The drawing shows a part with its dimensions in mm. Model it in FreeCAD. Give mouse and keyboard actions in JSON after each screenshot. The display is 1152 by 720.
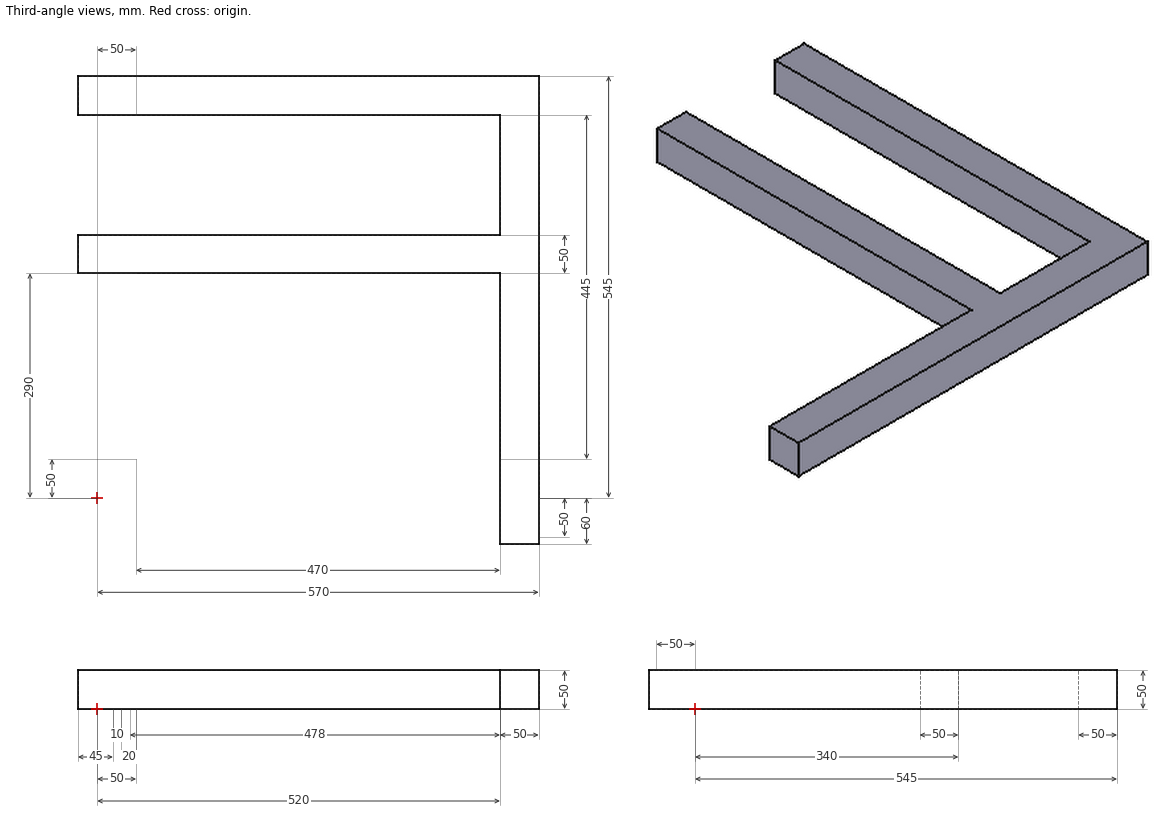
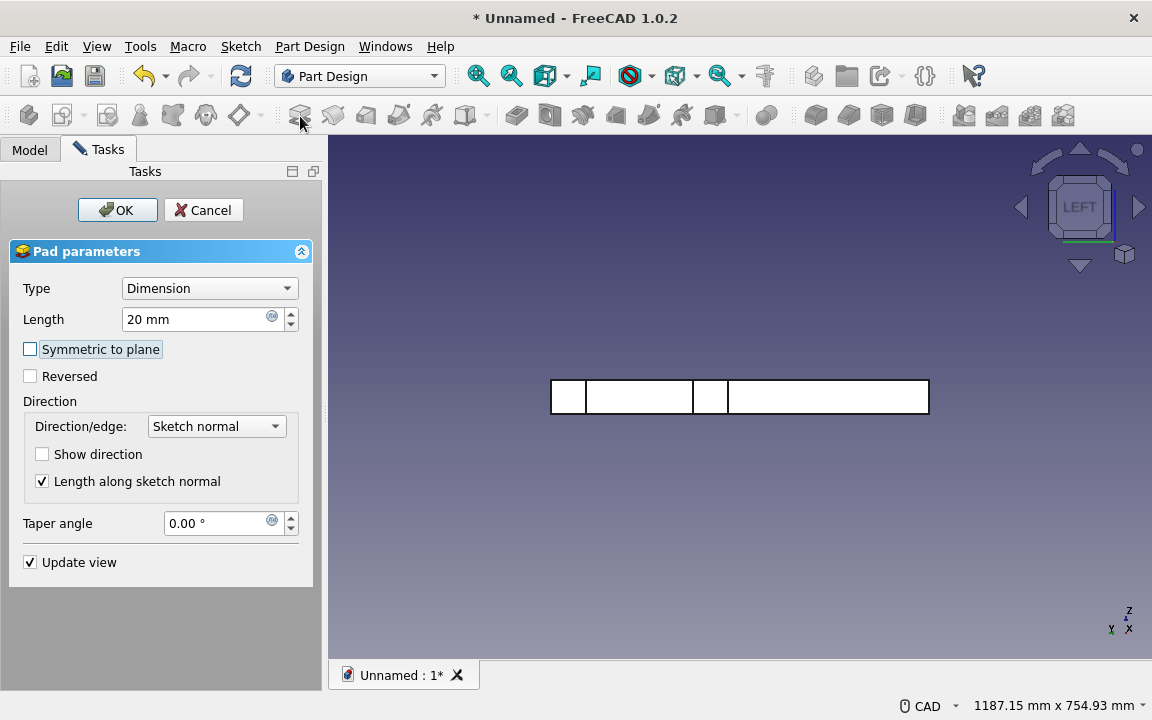
{"action": "left_click", "coordinate": [118, 210]}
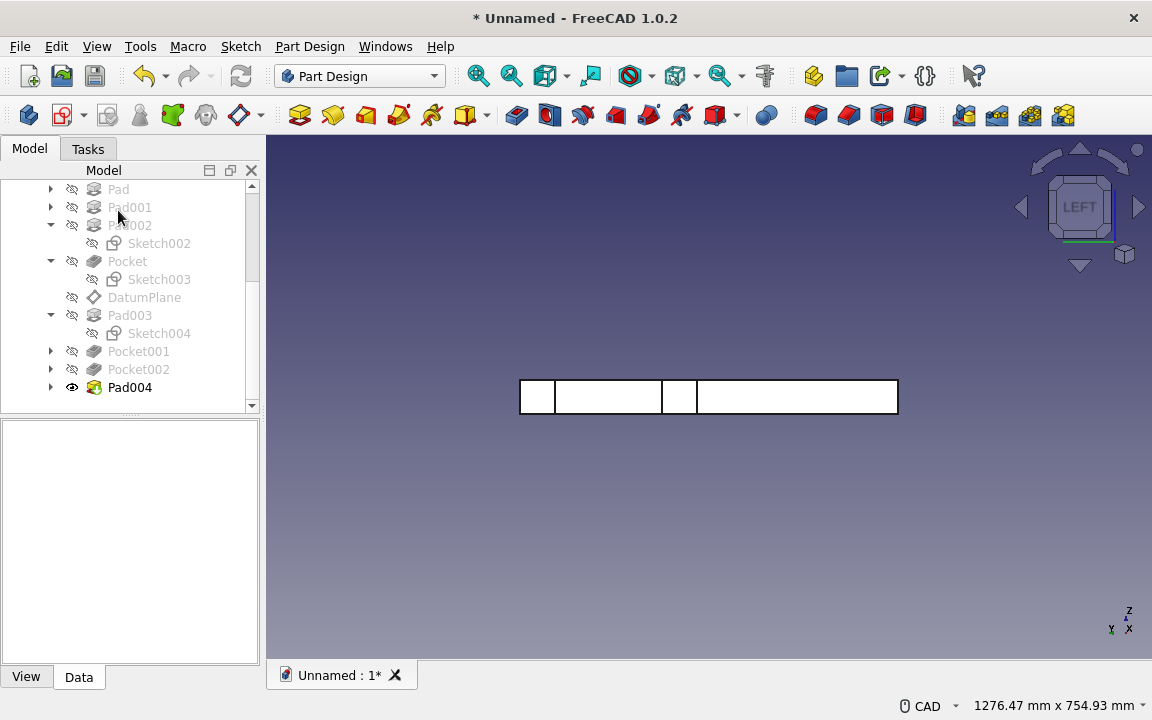
{"action": "key", "text": "v f"}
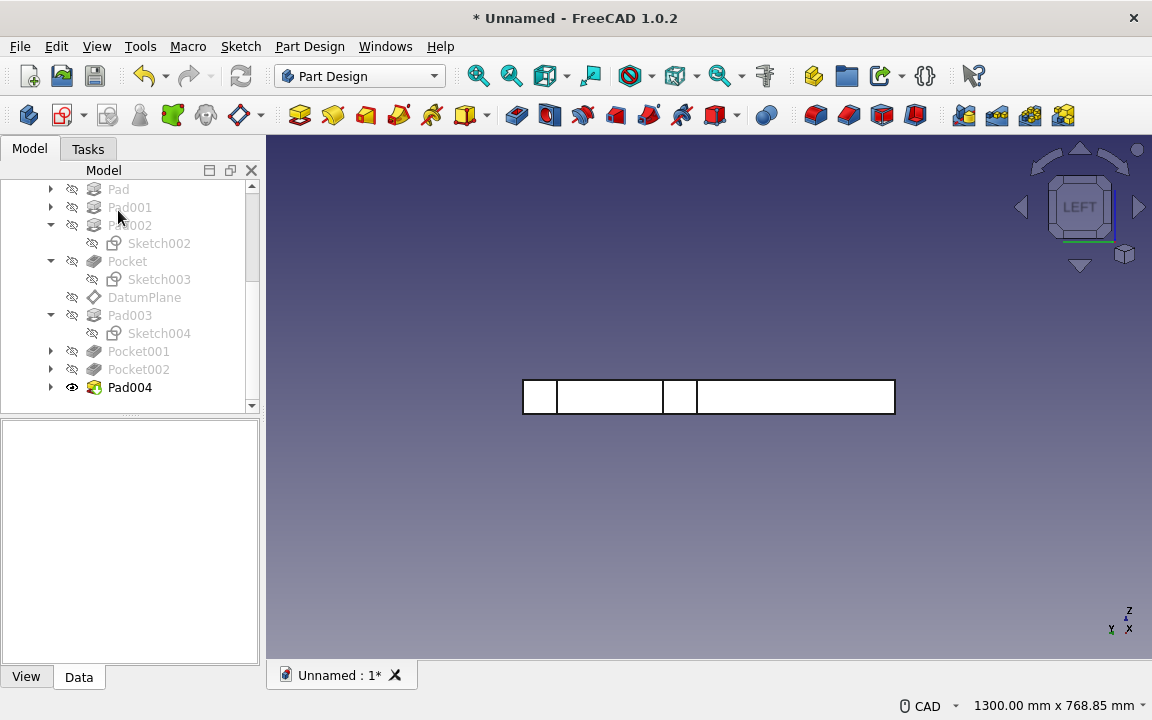
{"action": "left_click", "coordinate": [540, 396]}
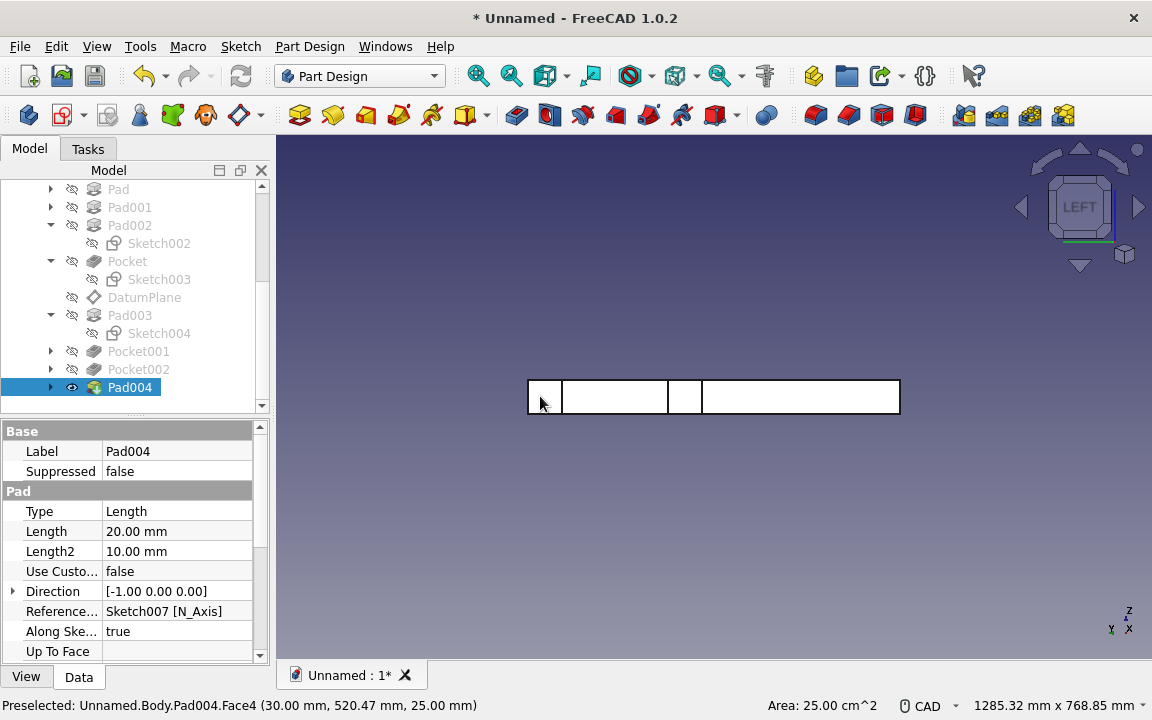
{"action": "left_click", "coordinate": [62, 116]}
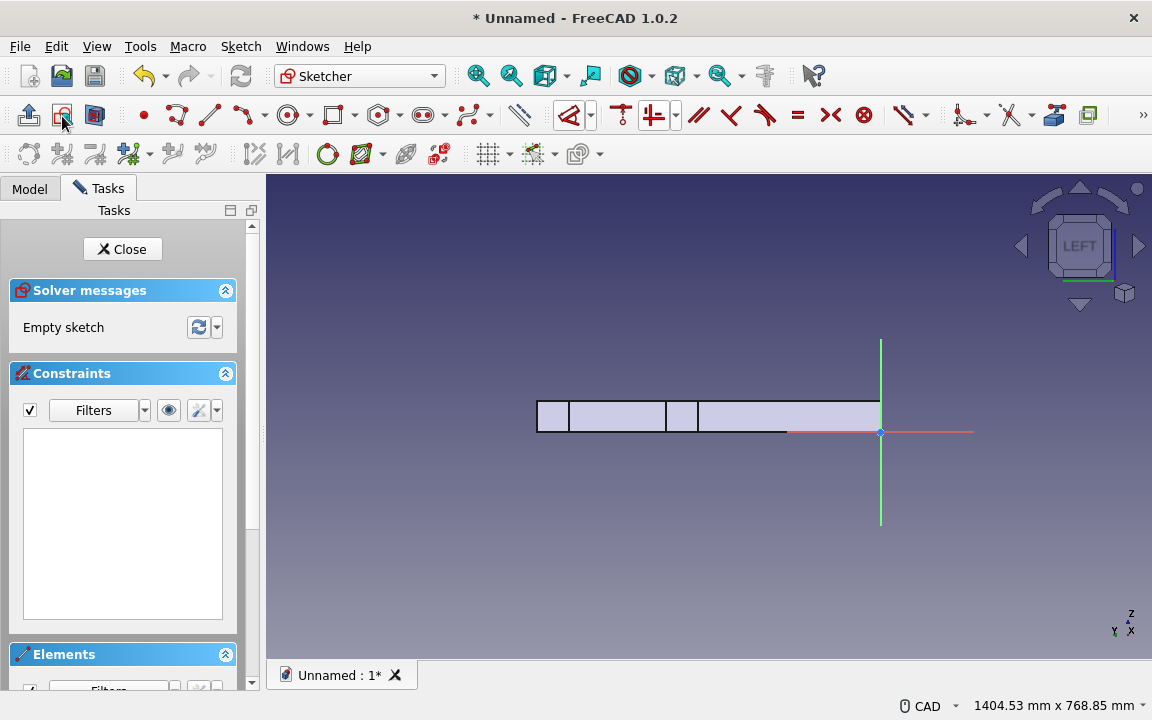
{"action": "scroll", "coordinate": [848, 416], "scroll_direction": "up", "scroll_amount": 2}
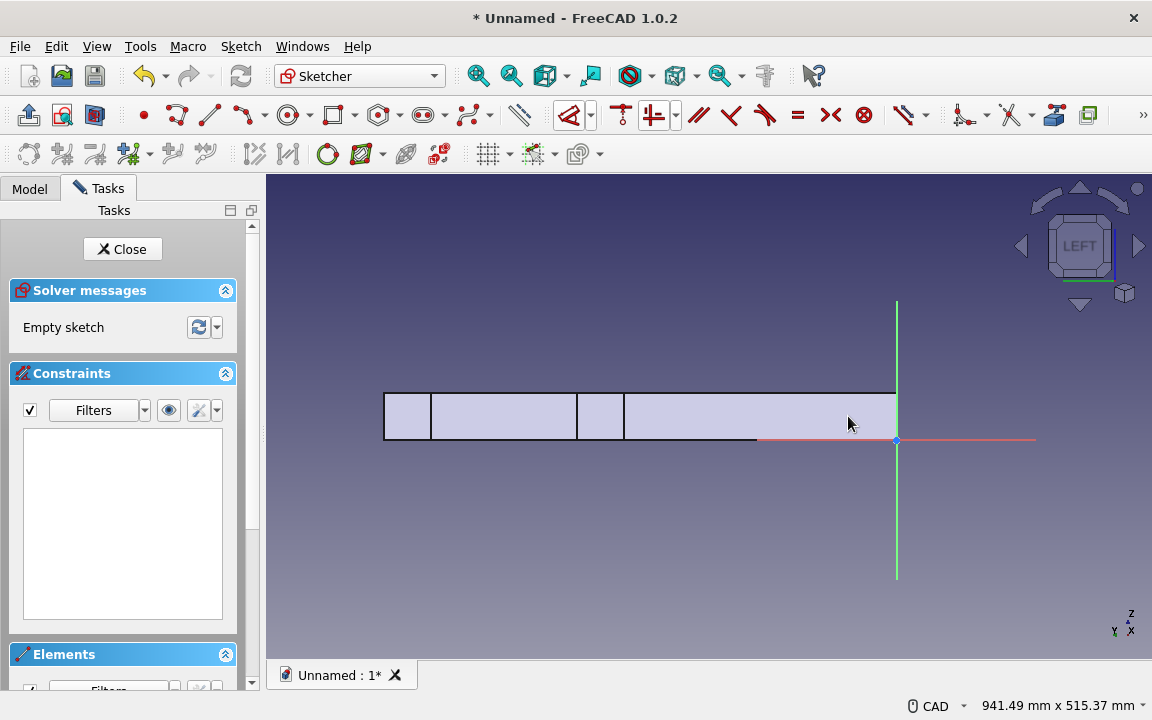
{"action": "key", "text": "g r"}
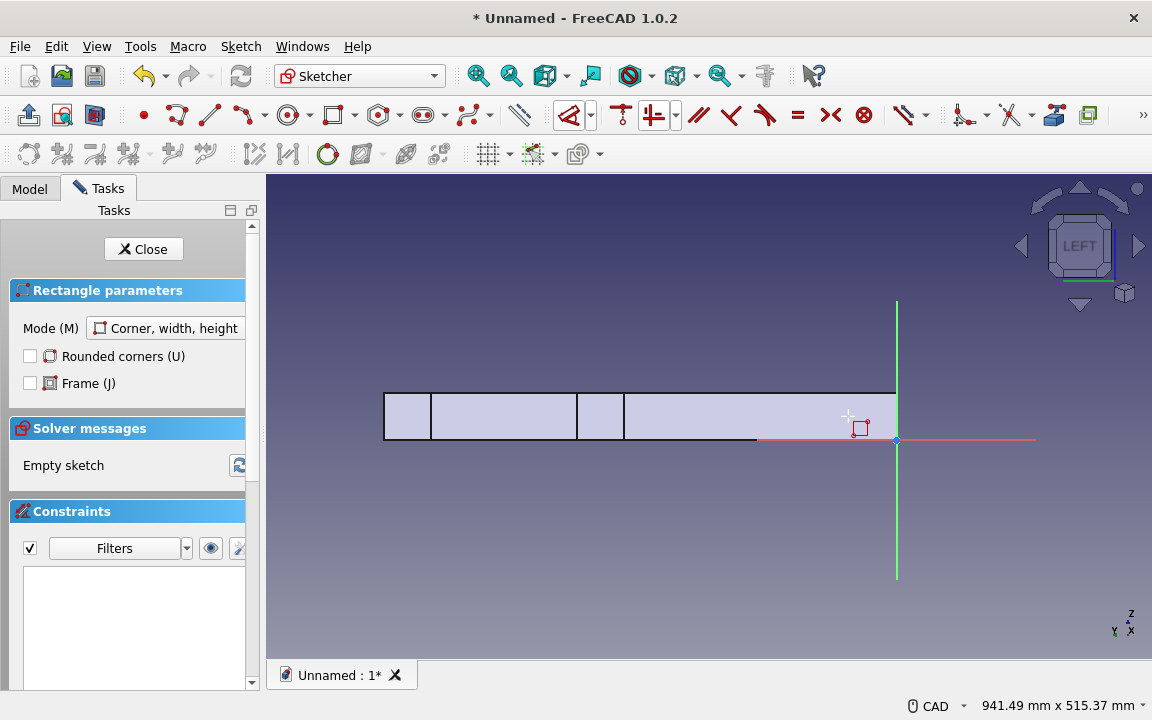
{"action": "left_click", "coordinate": [384, 393]}
{"action": "left_click", "coordinate": [431, 440]}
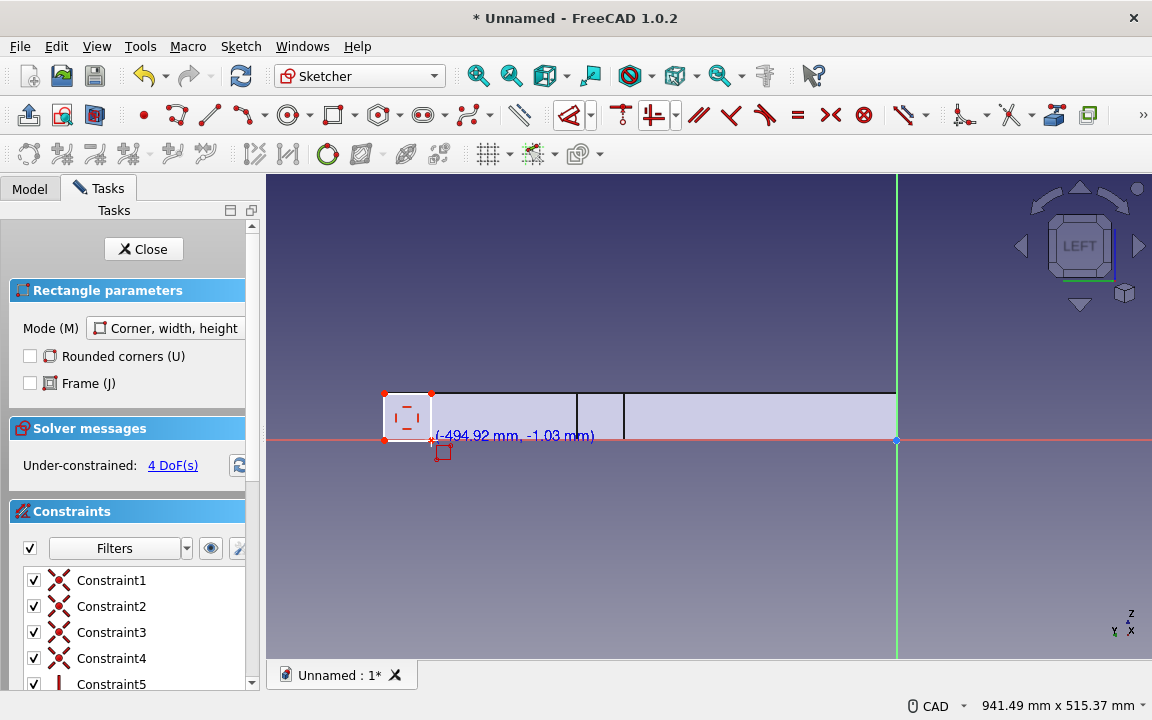
{"action": "left_click", "coordinate": [577, 393]}
{"action": "left_click", "coordinate": [624, 440]}
{"action": "key", "text": "Escape"}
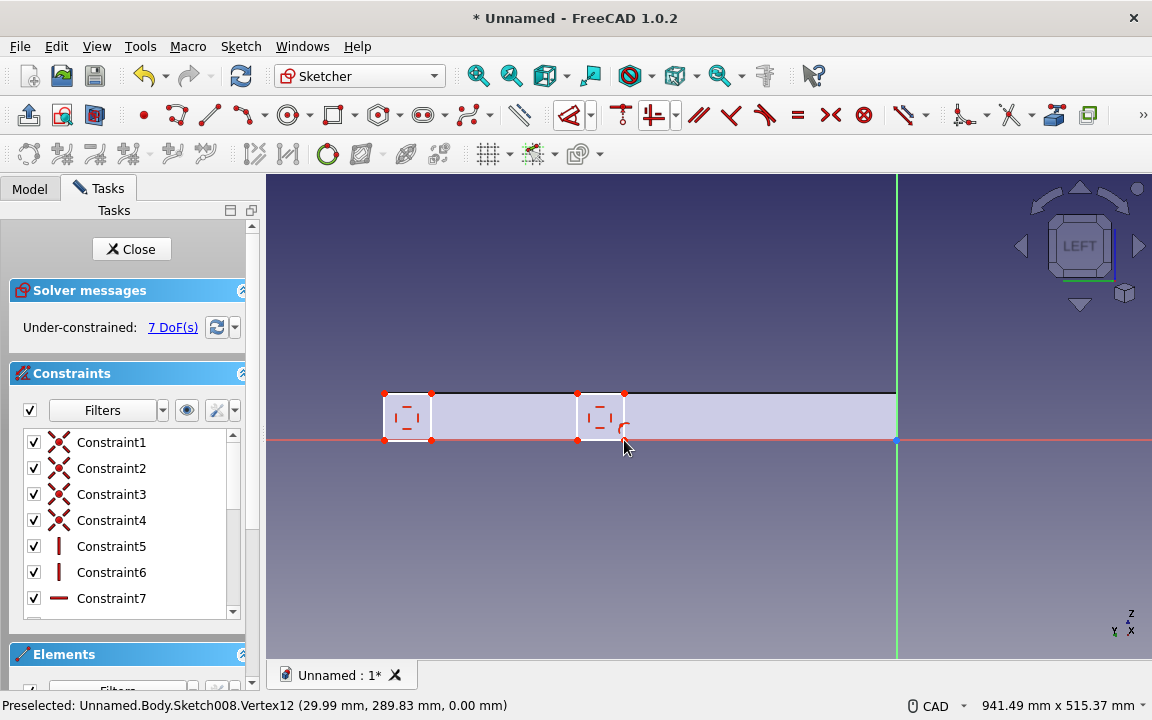
{"action": "left_click", "coordinate": [384, 441]}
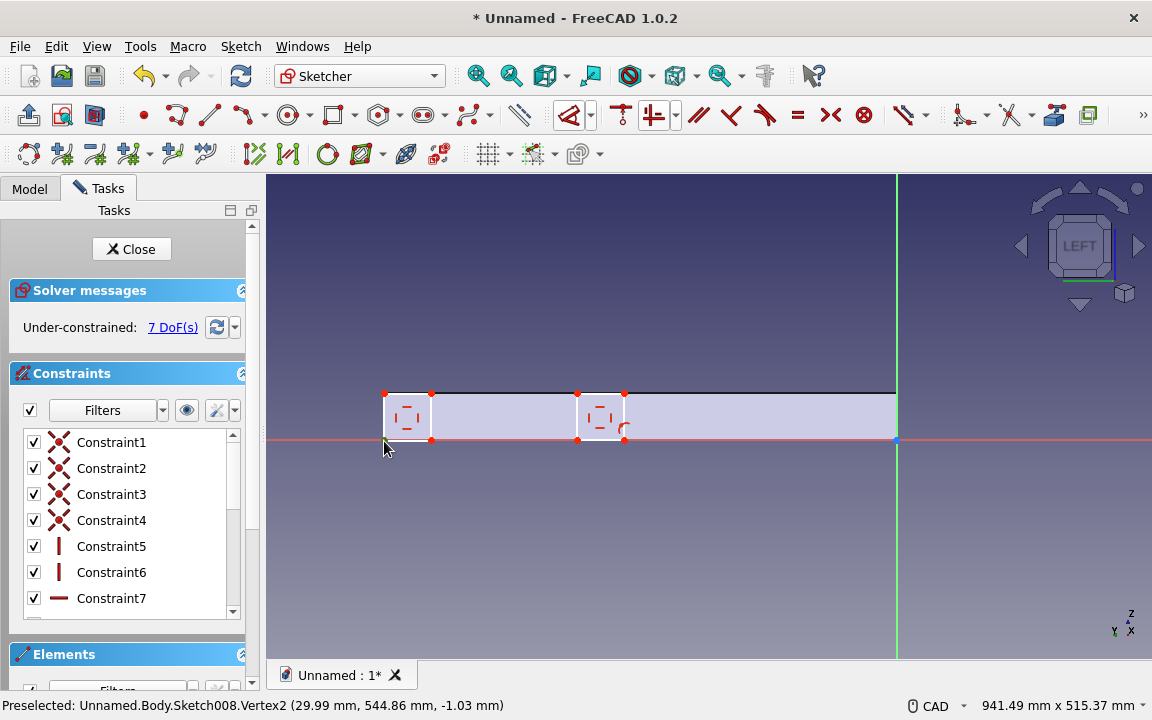
{"action": "left_click", "coordinate": [344, 440]}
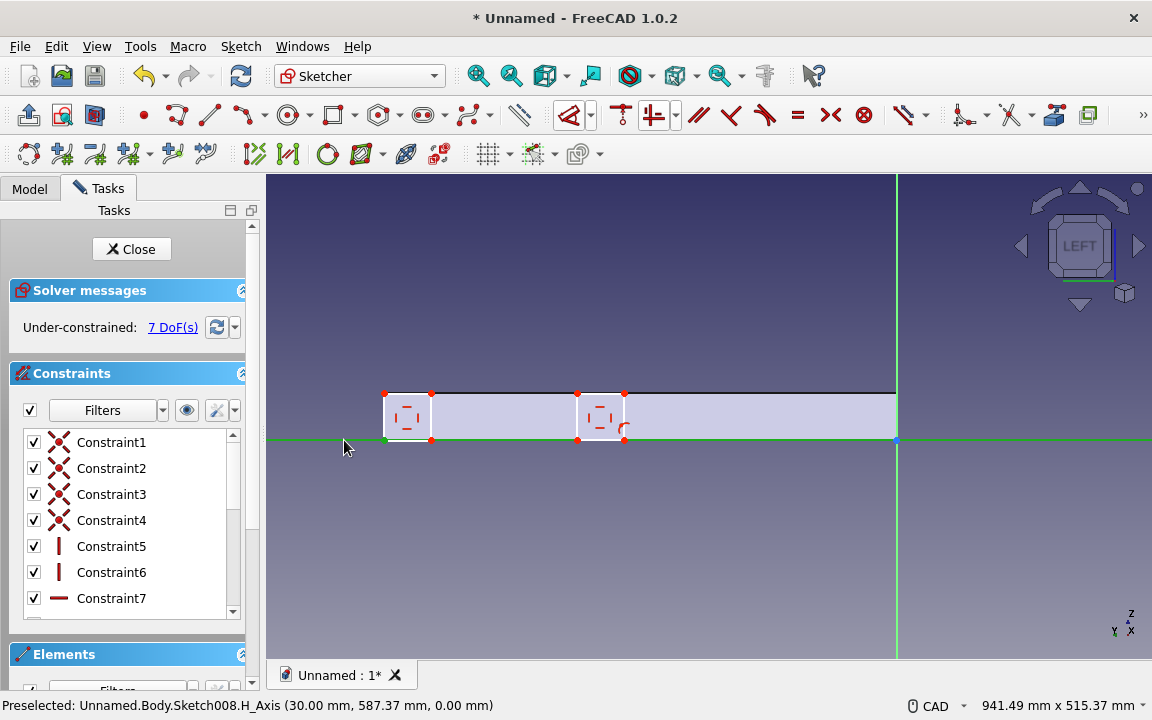
{"action": "key", "text": "c"}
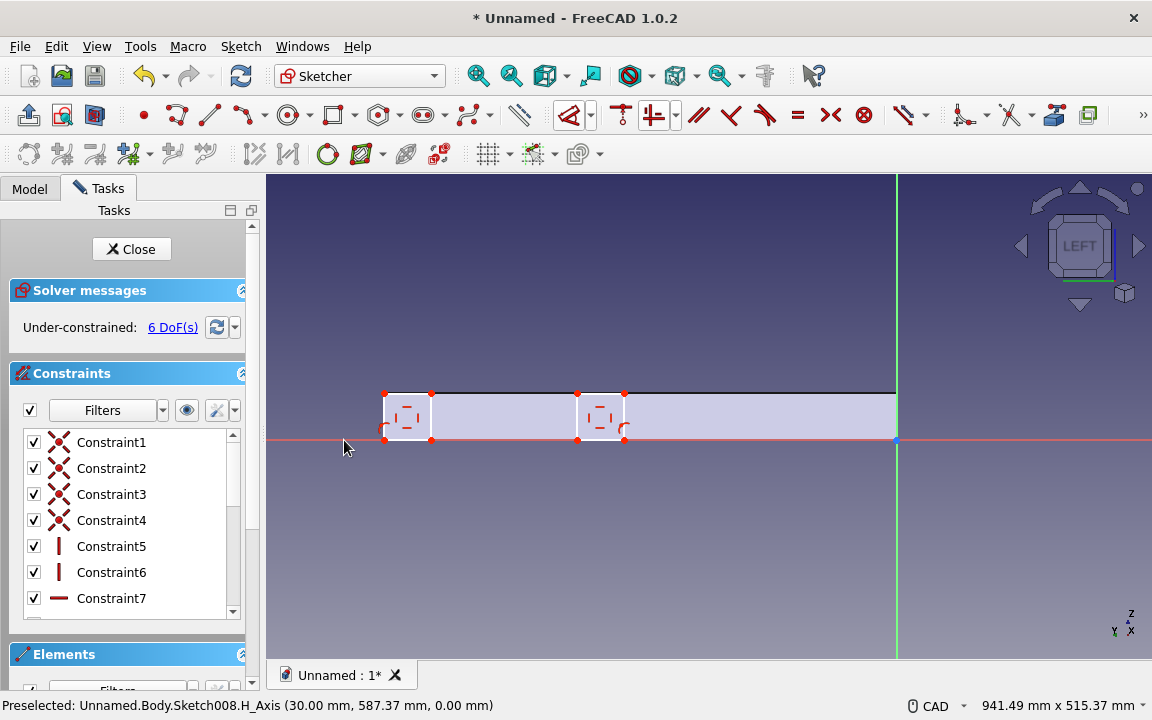
{"action": "left_click", "coordinate": [384, 408]}